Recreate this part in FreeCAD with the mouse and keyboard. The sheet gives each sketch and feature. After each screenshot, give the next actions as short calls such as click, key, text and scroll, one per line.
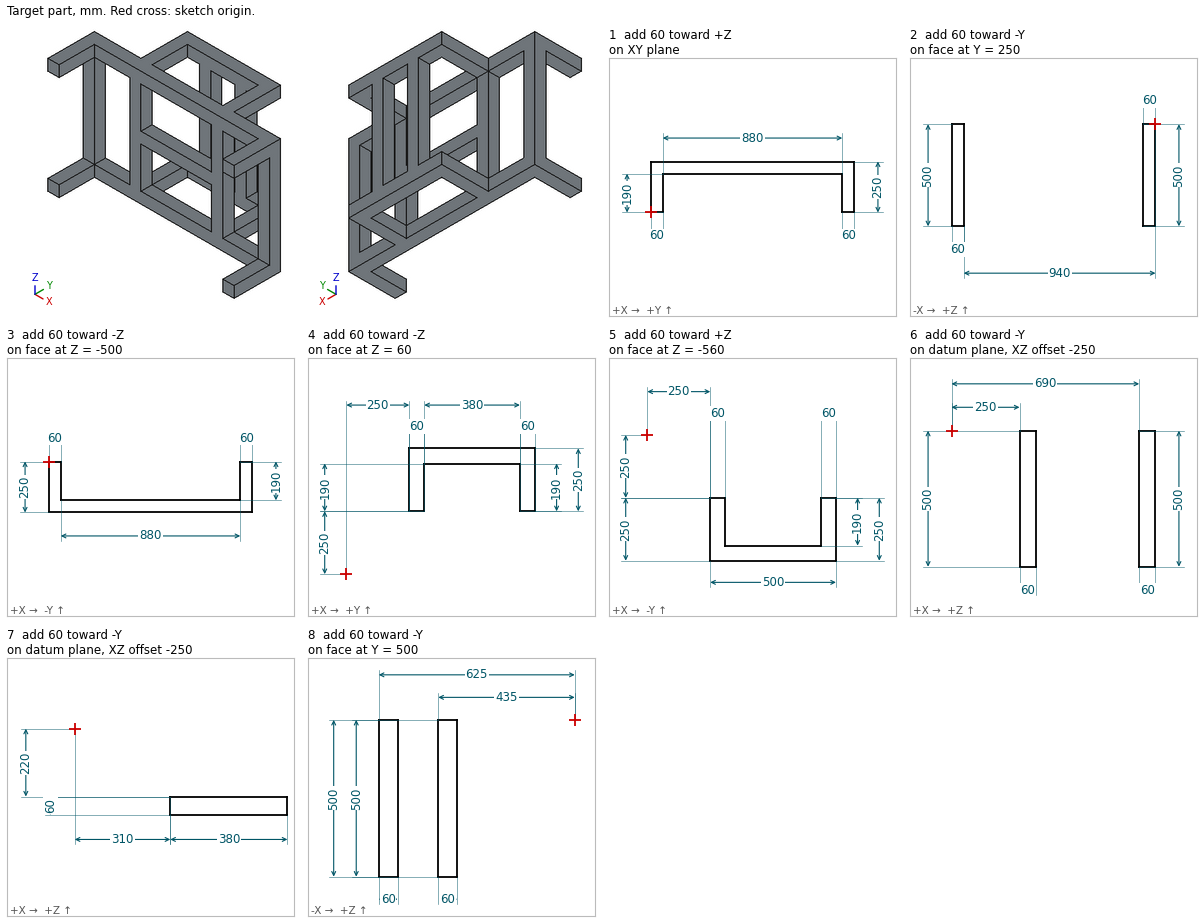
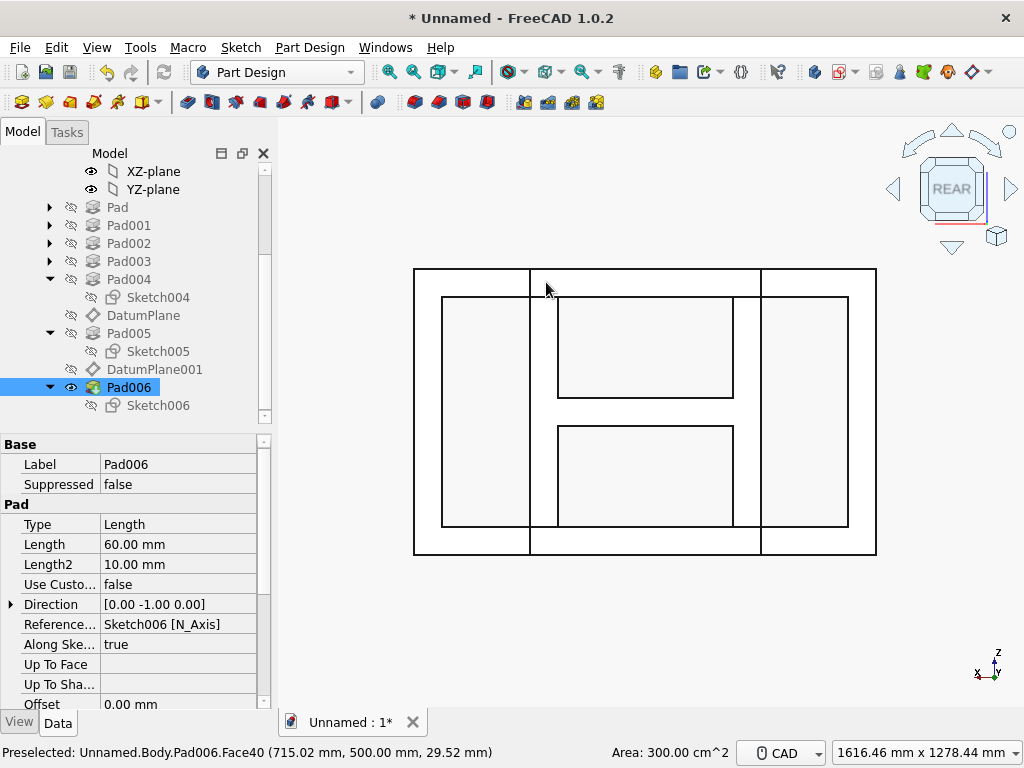
click(840, 72)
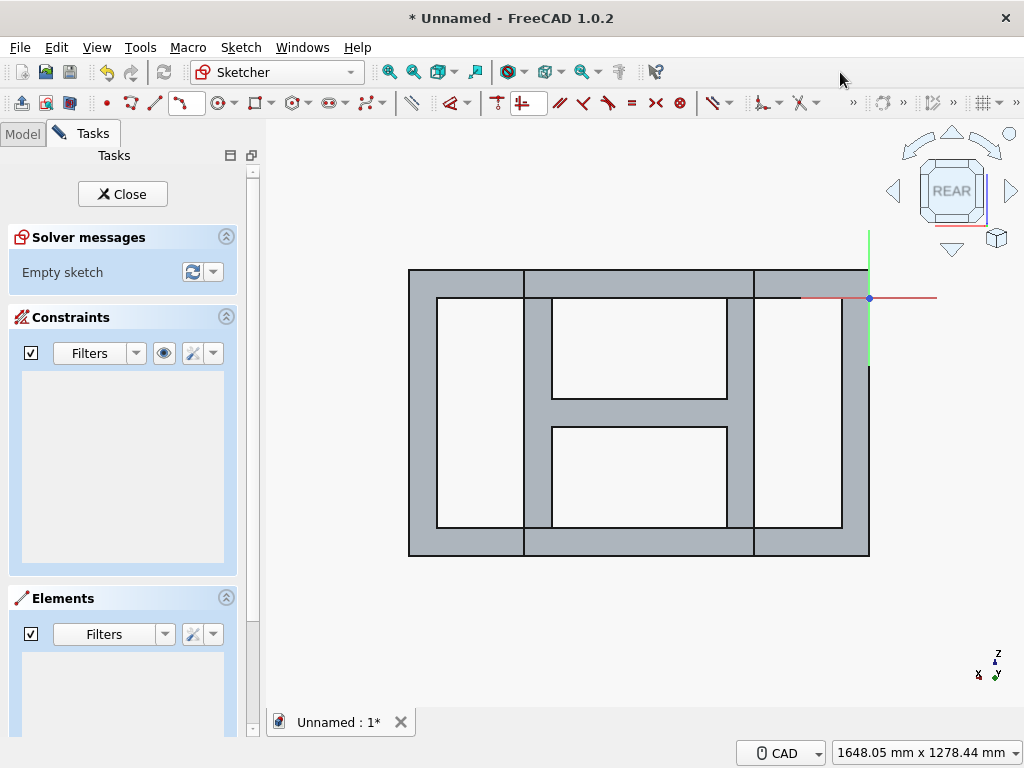
scroll(294, 413, down, 1)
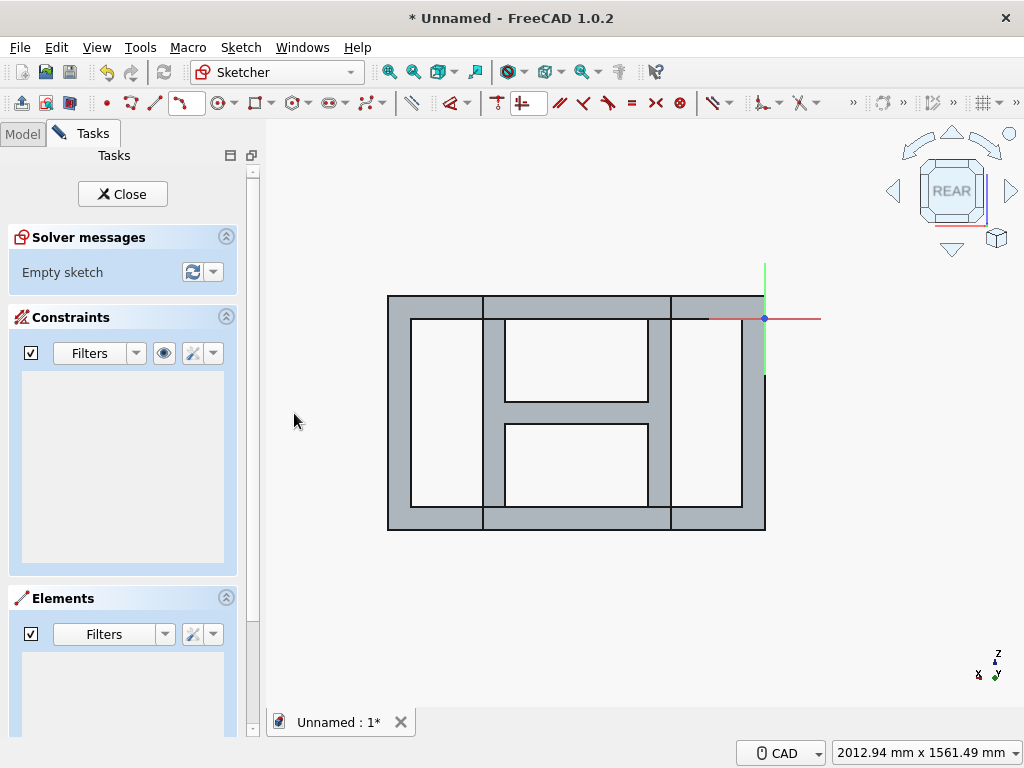
scroll(733, 413, up, 3)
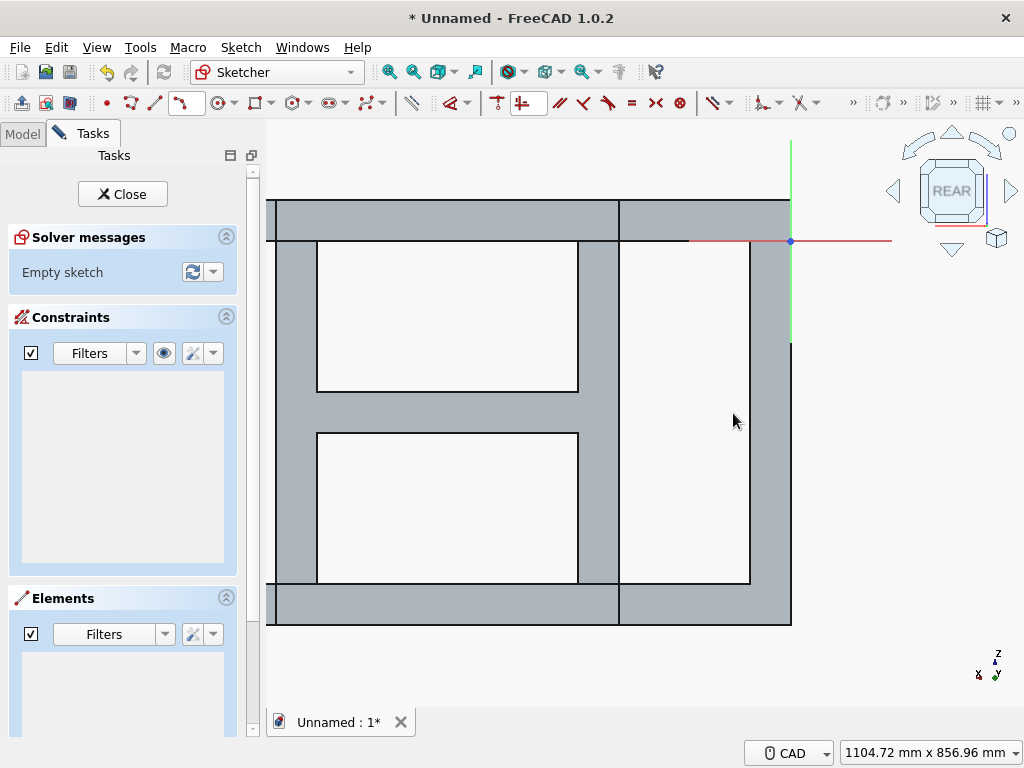
click(256, 104)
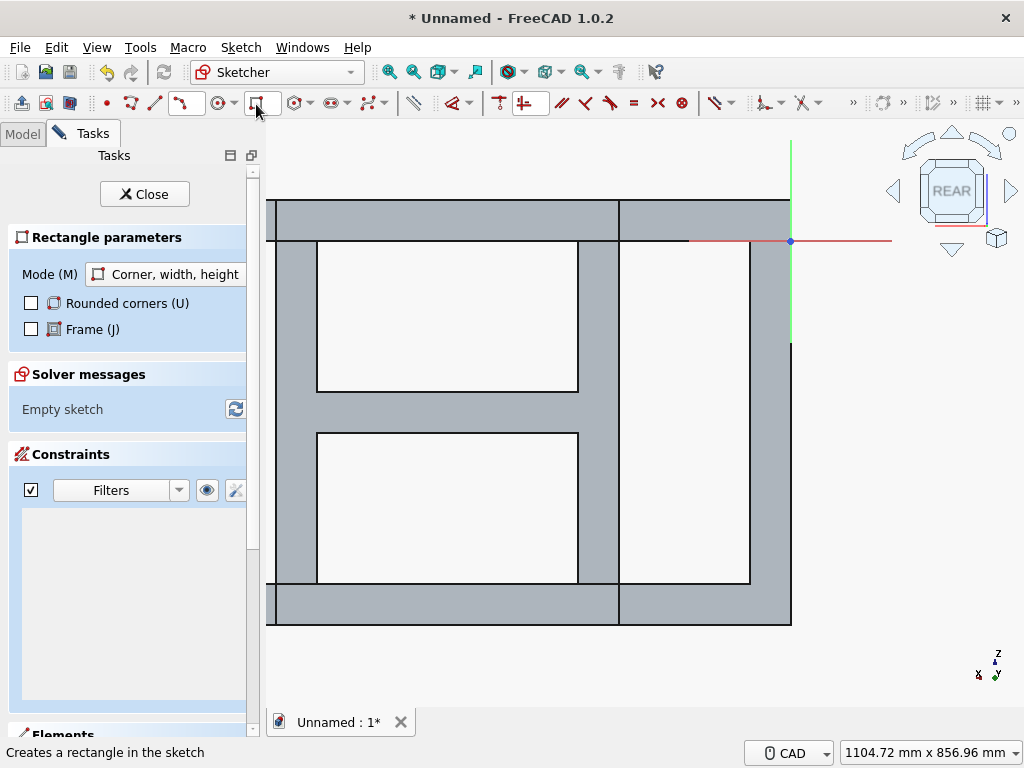
click(492, 241)
click(533, 584)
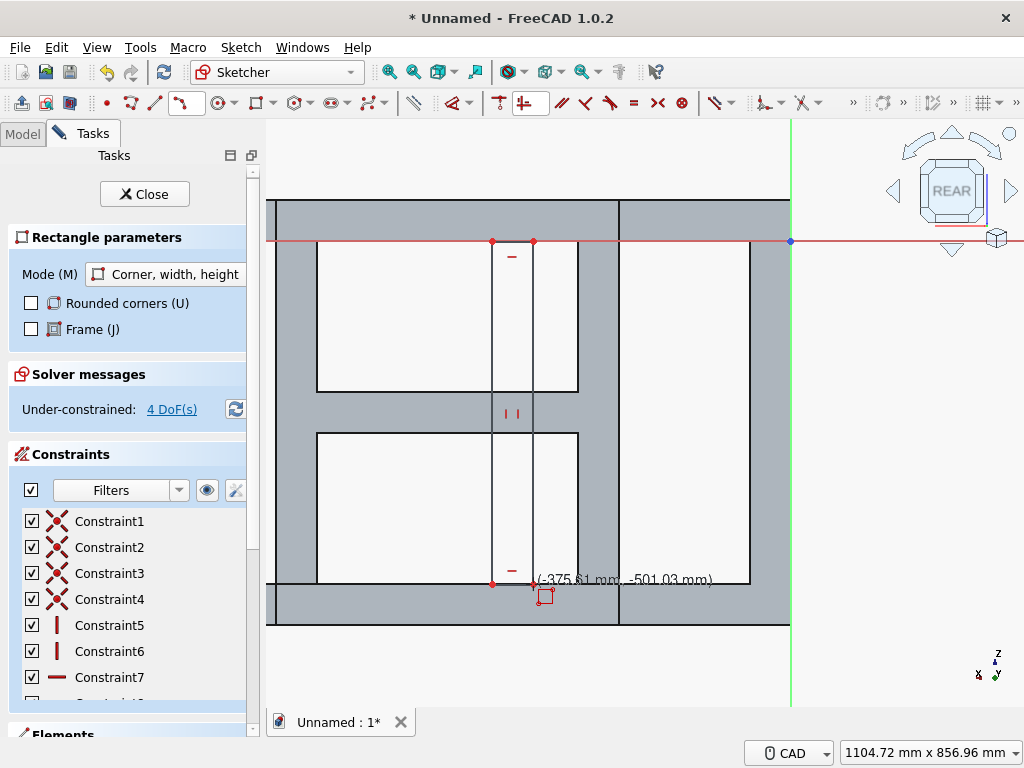
click(362, 241)
click(403, 584)
key(Escape)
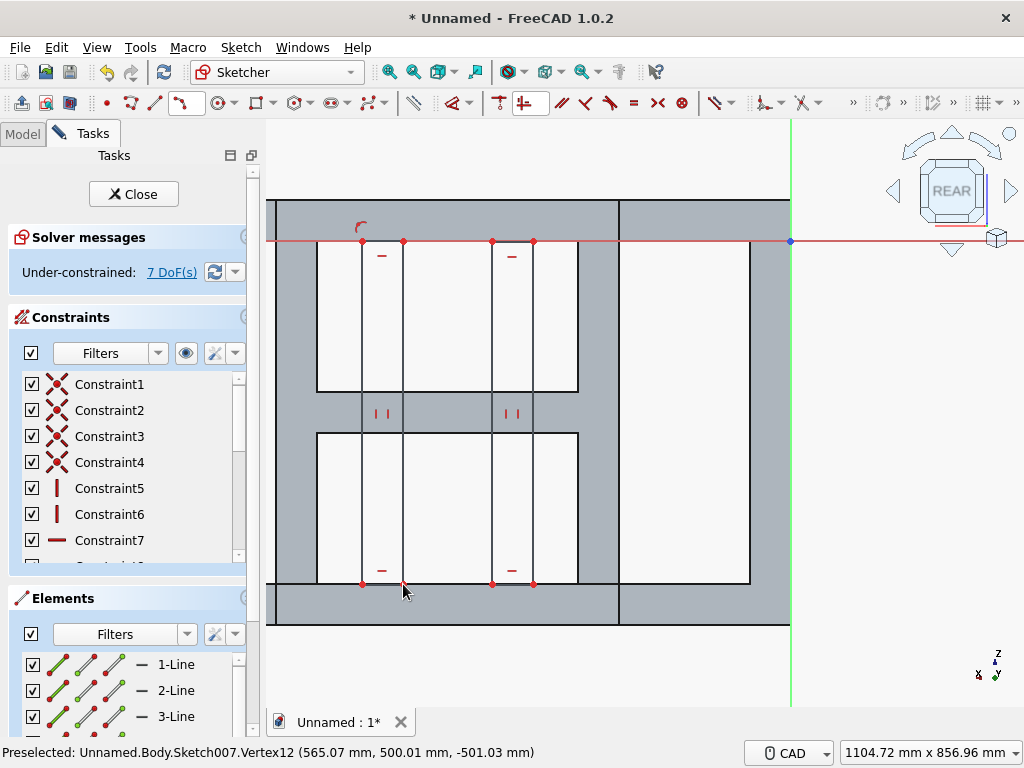
click(492, 242)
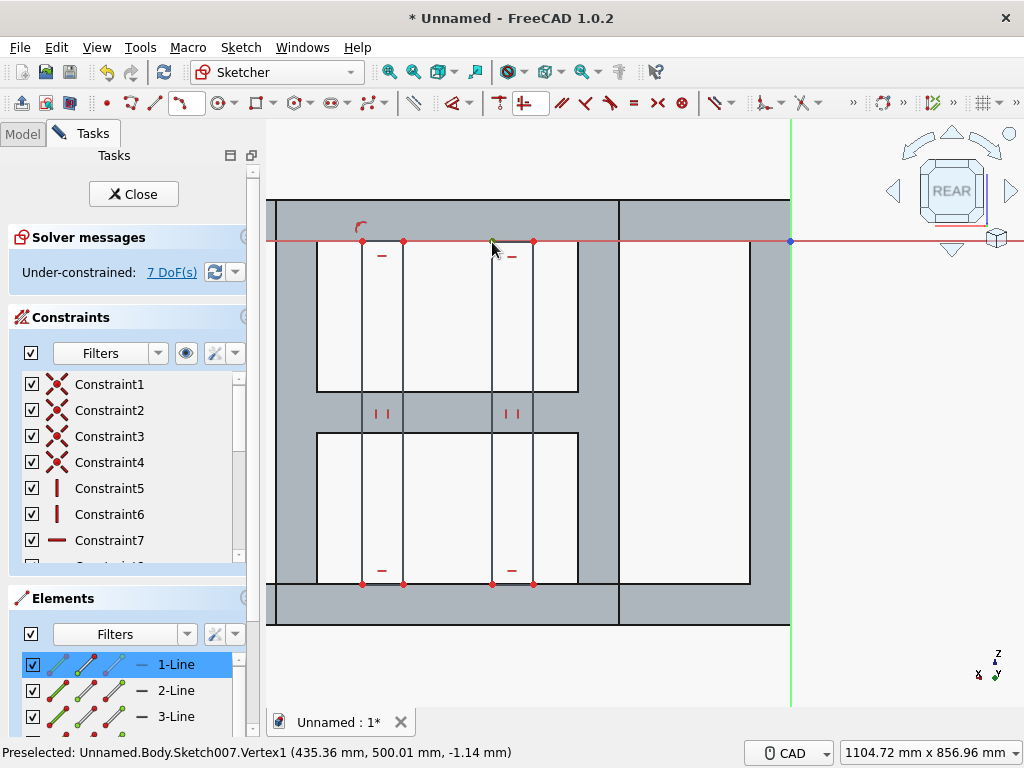
click(455, 241)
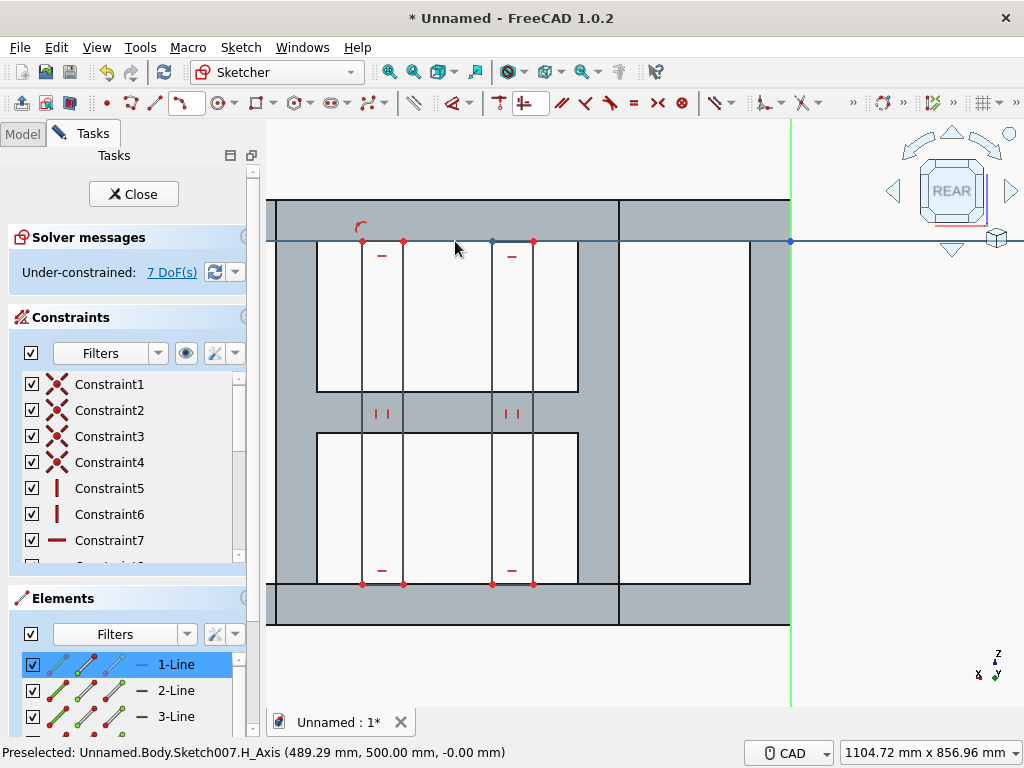
click(500, 104)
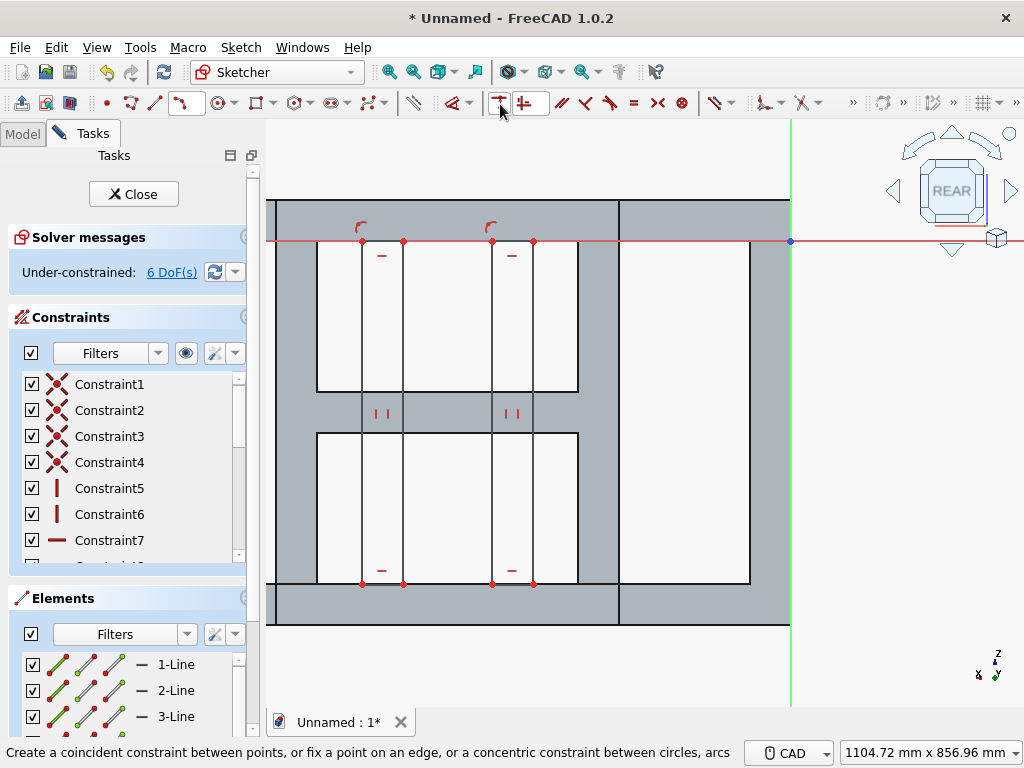
click(452, 104)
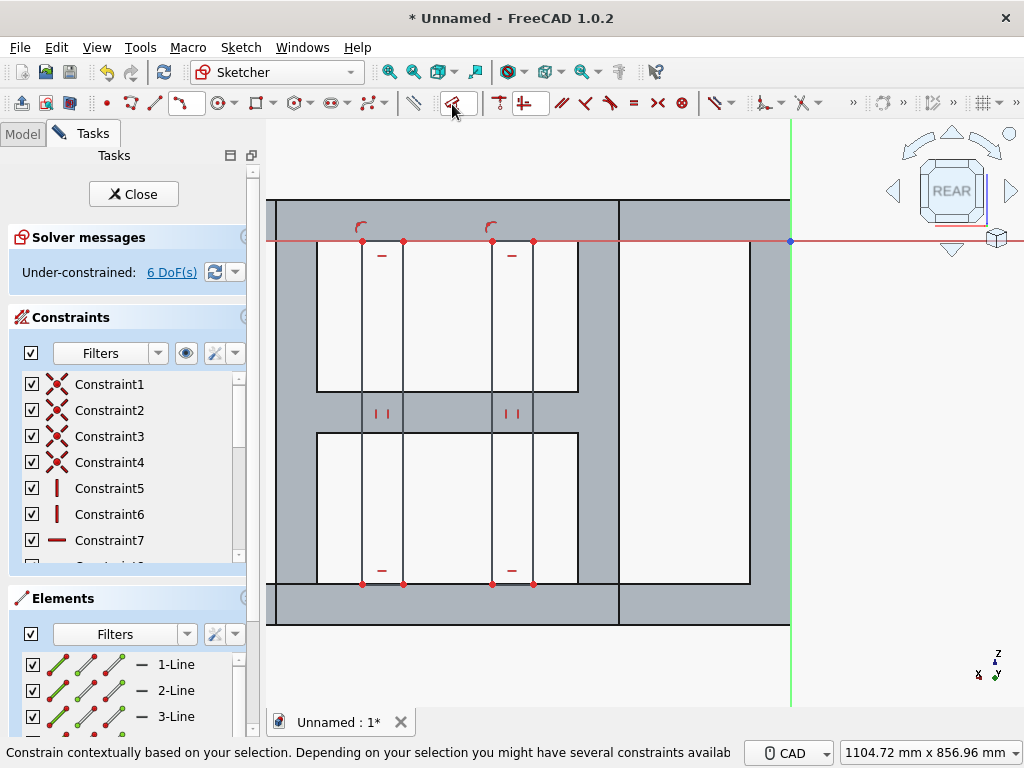
click(504, 585)
click(513, 619)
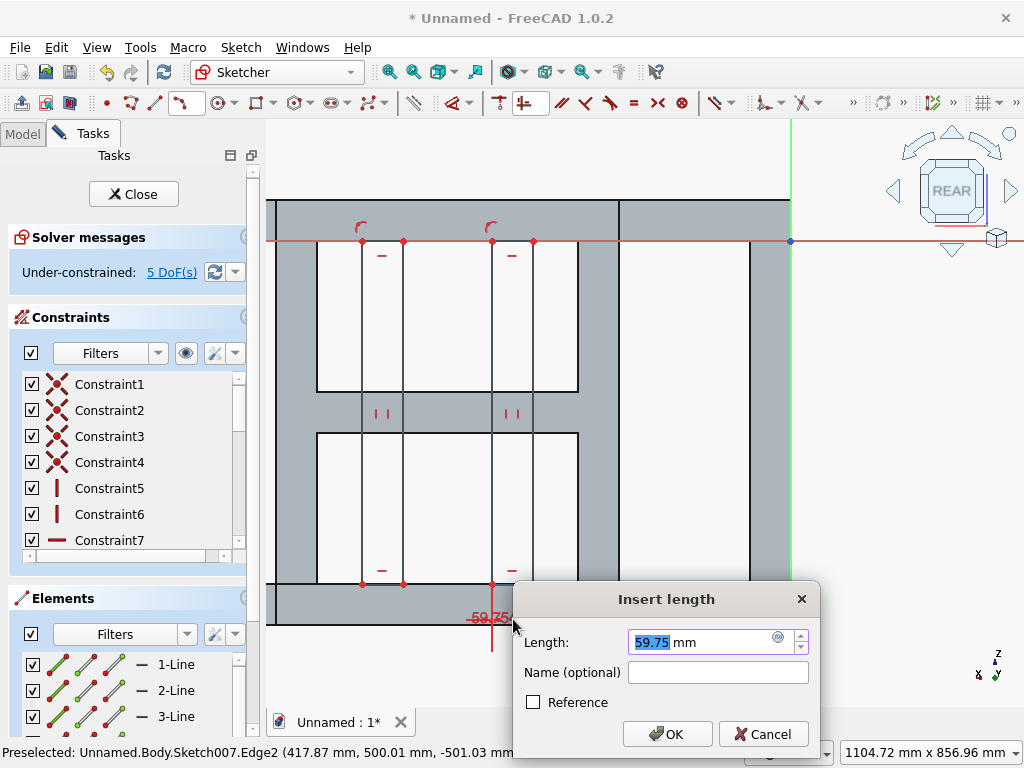
text(60)
key(Return)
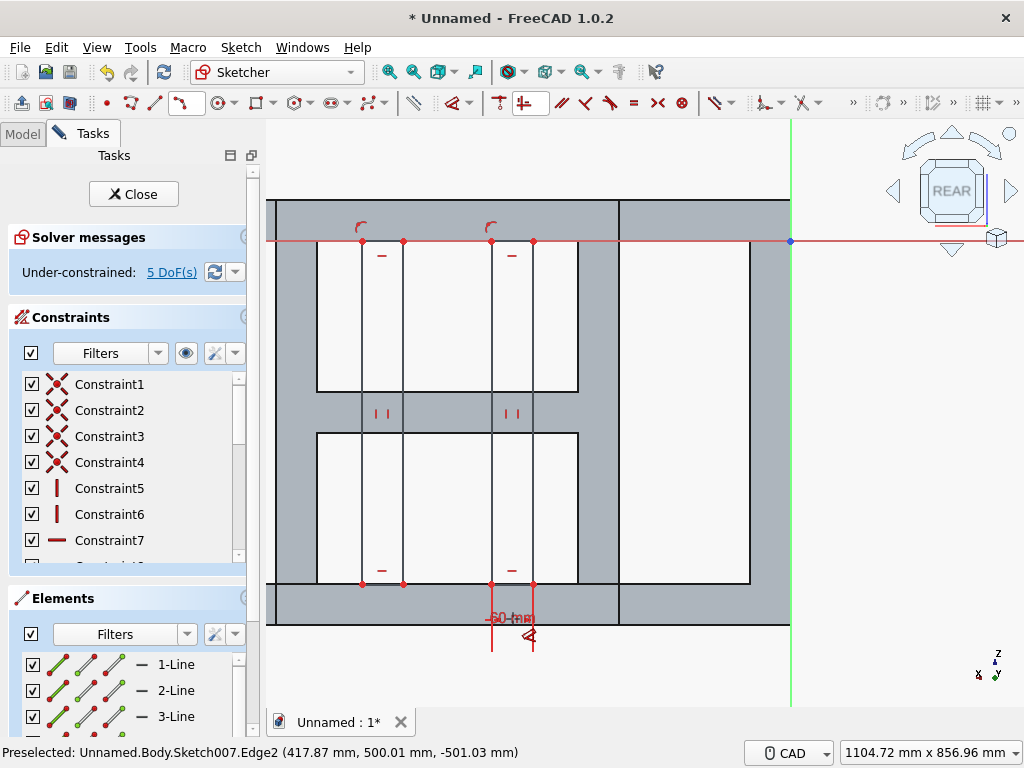
click(374, 585)
click(383, 619)